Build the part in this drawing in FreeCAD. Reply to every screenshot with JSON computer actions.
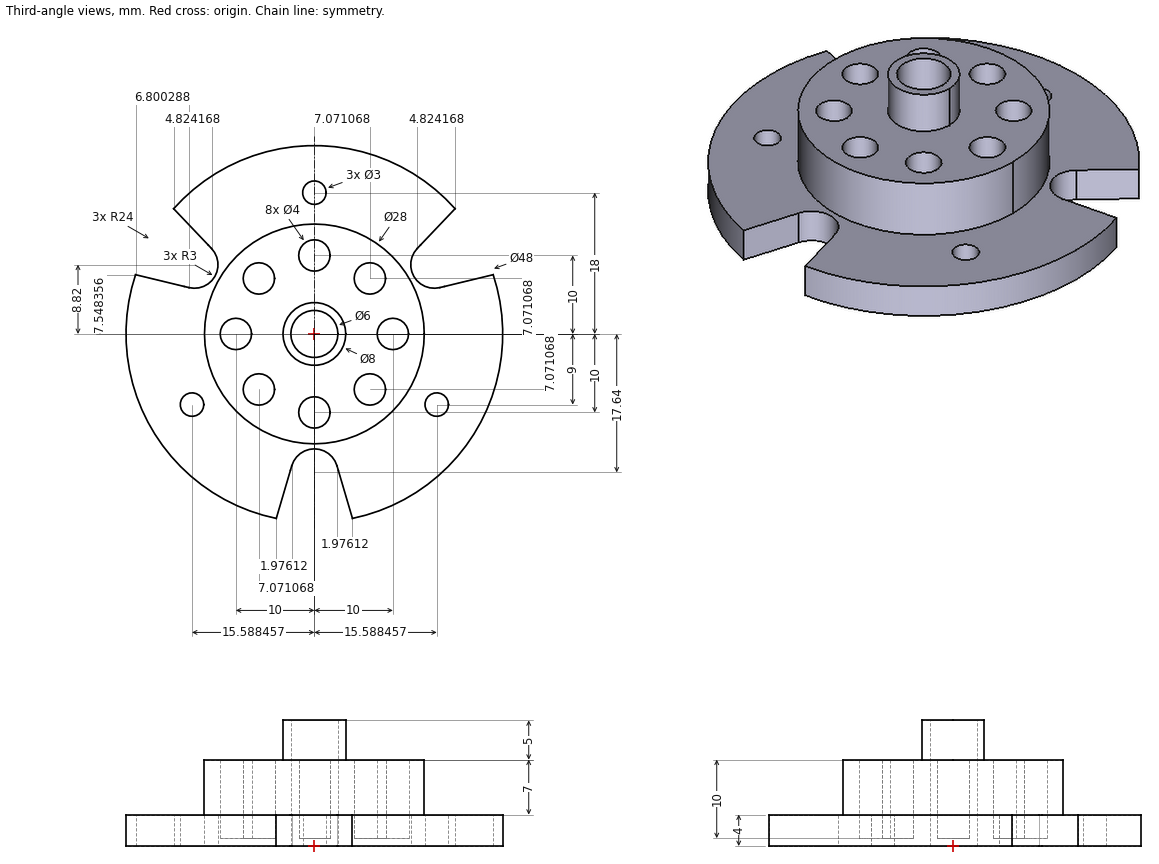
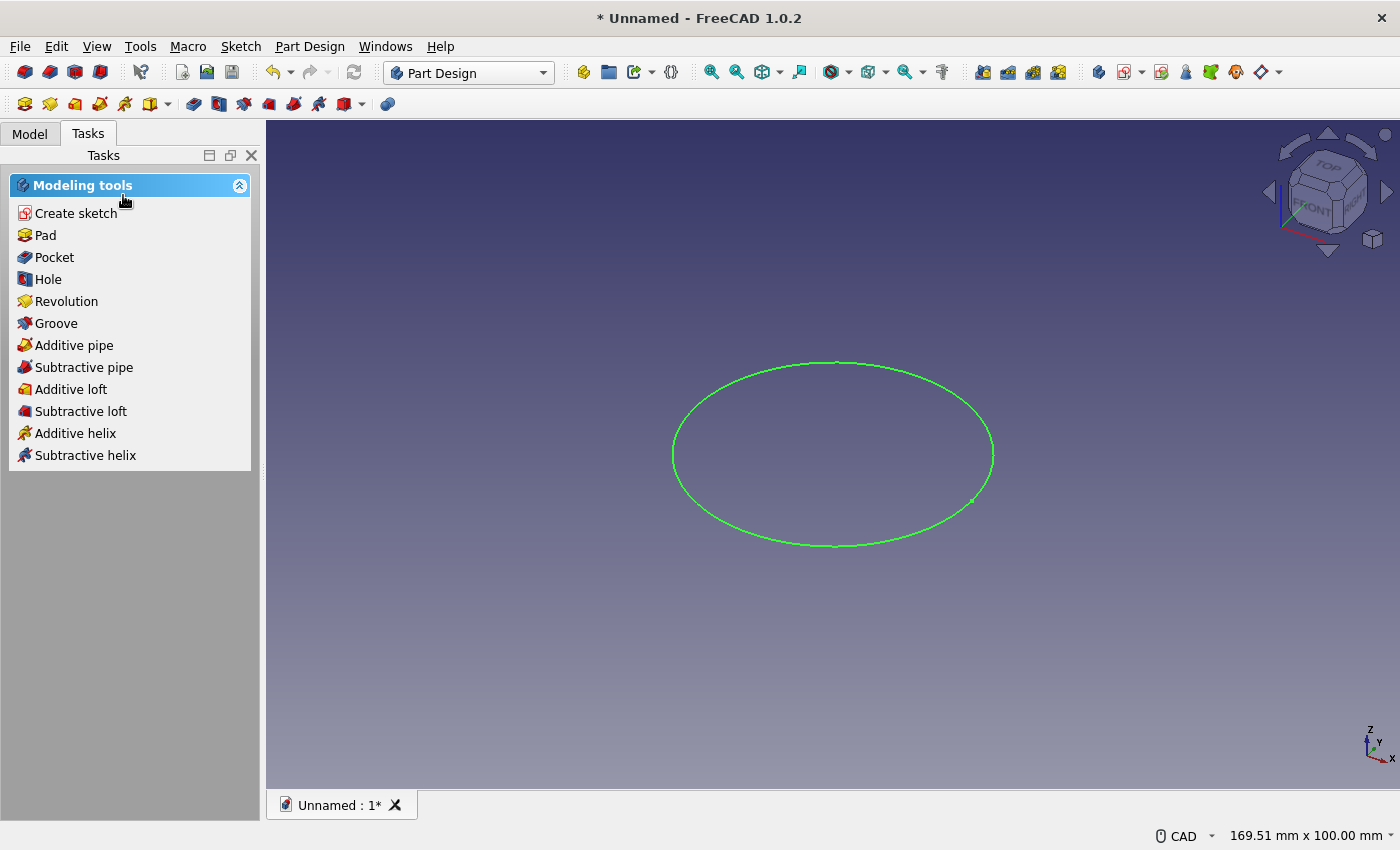
{"action": "left_click", "coordinate": [25, 104]}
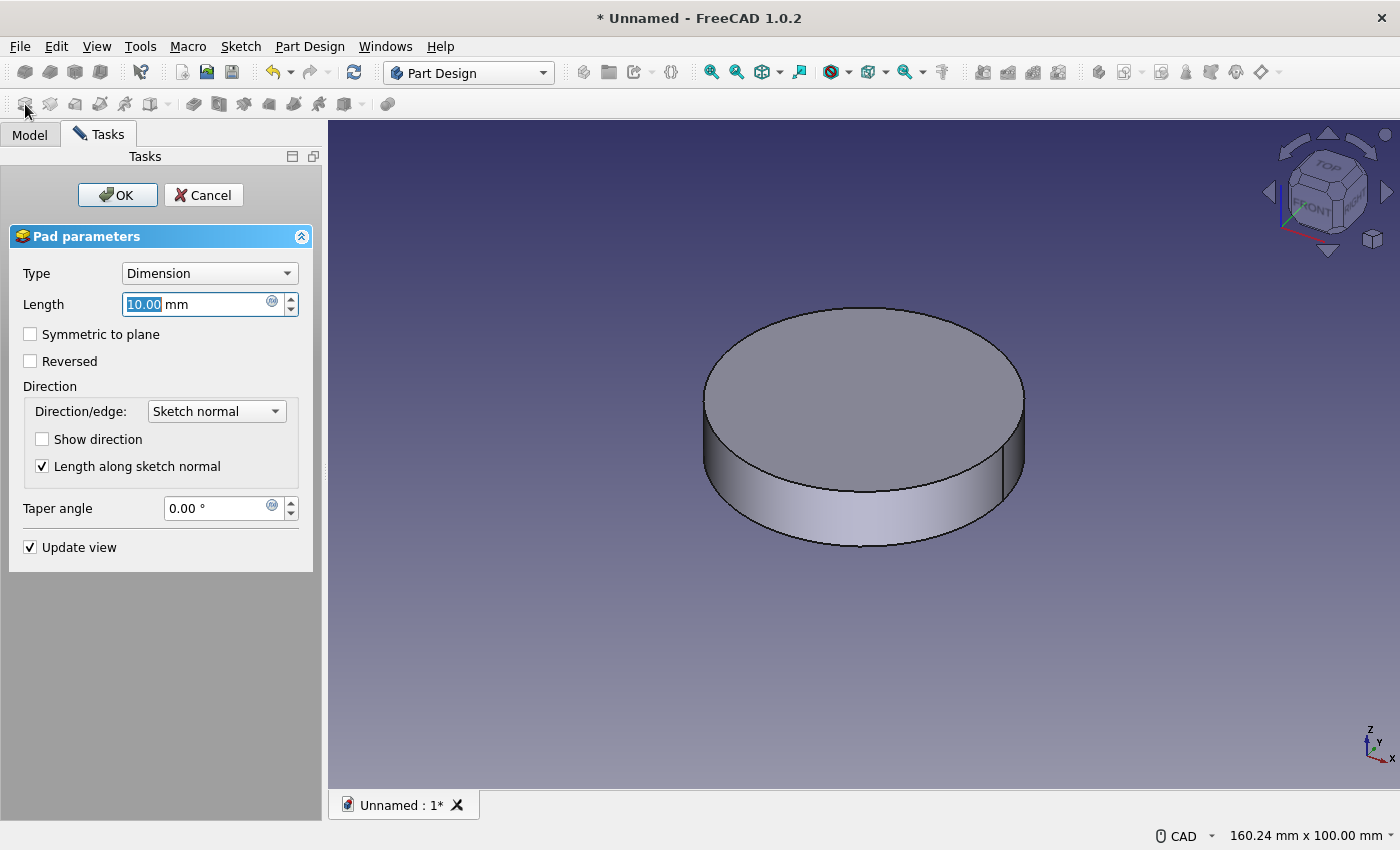
{"action": "type", "text": "4"}
{"action": "key", "text": "Tab"}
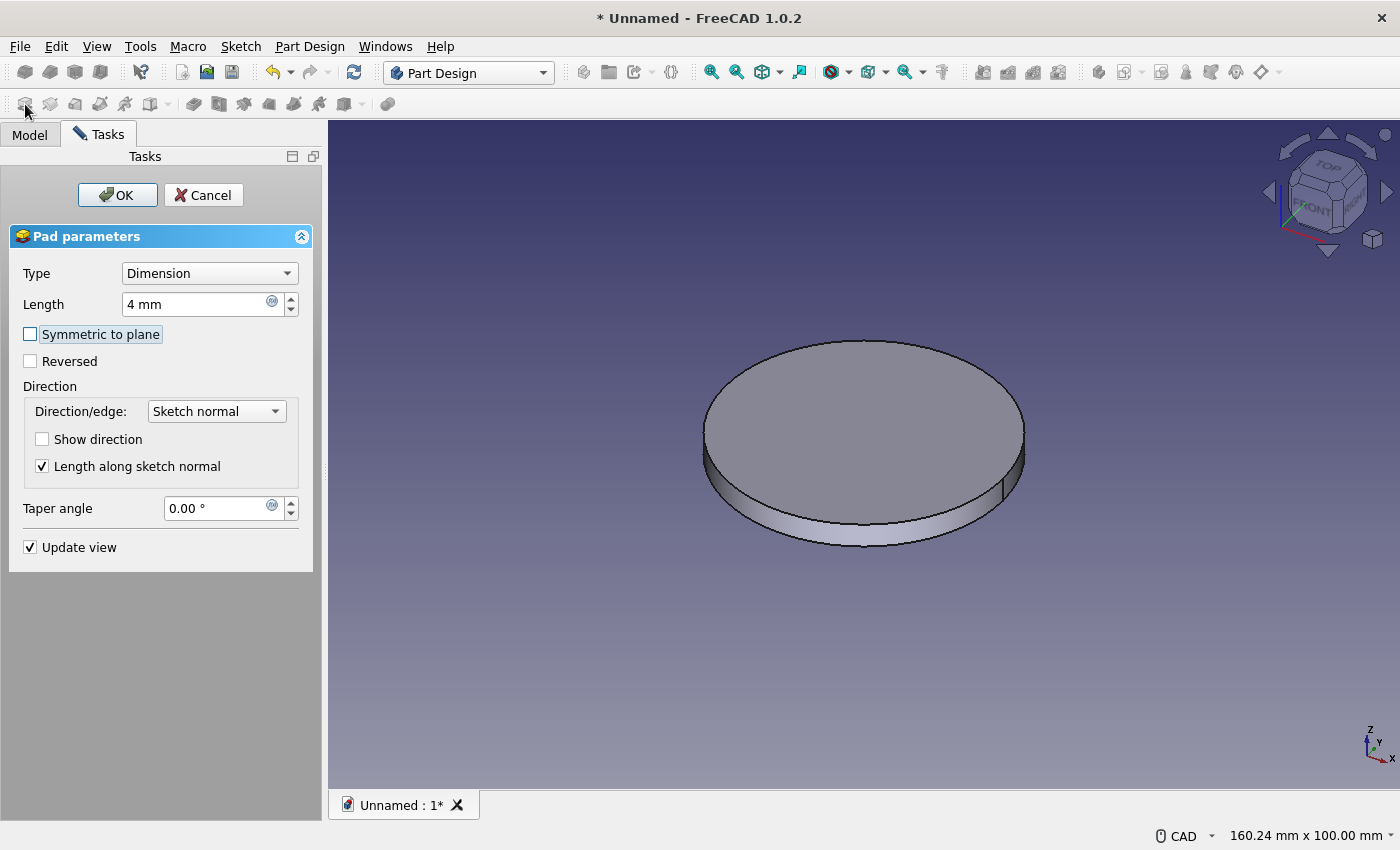
{"action": "left_click", "coordinate": [118, 195]}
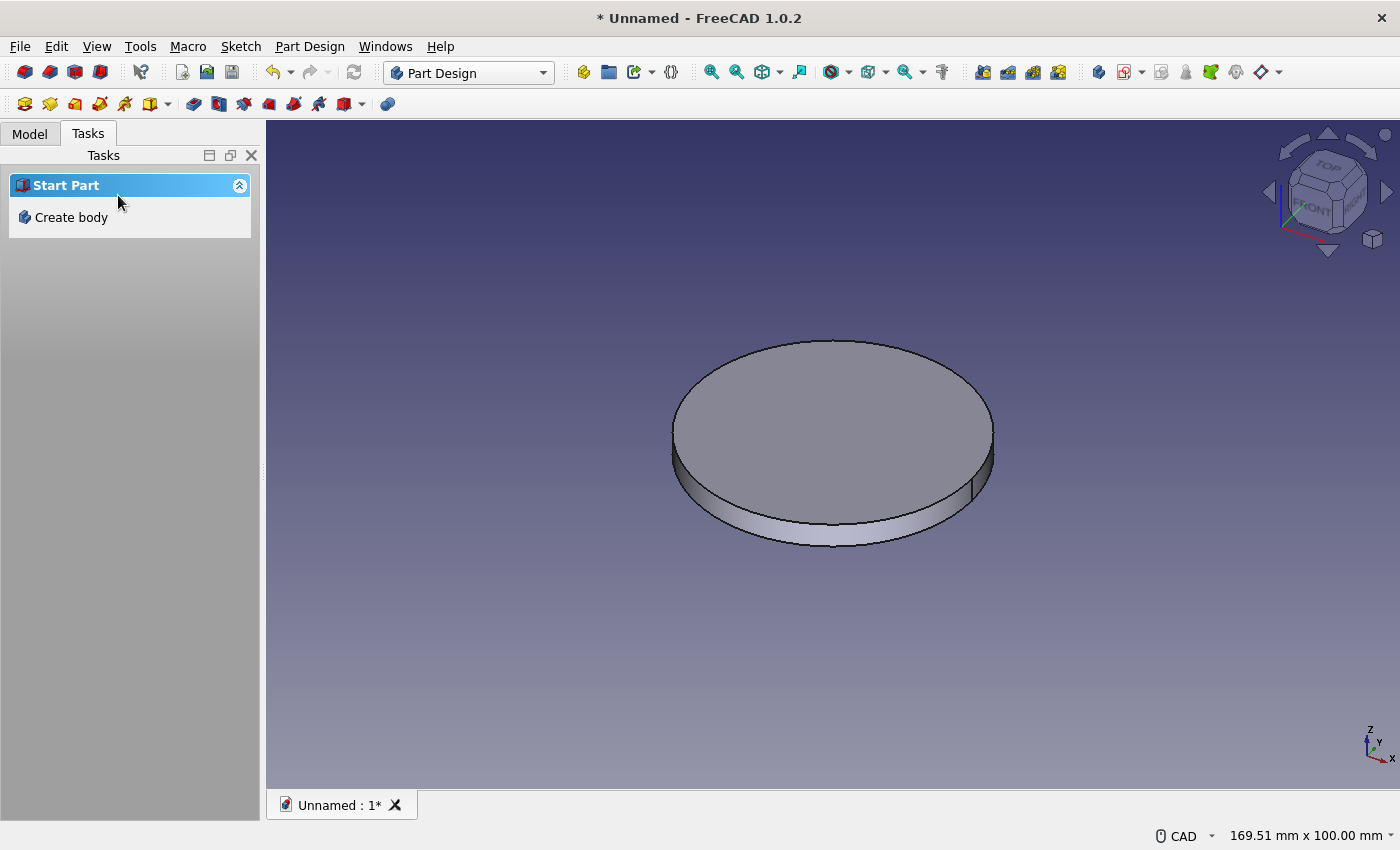
{"action": "key", "text": "v f"}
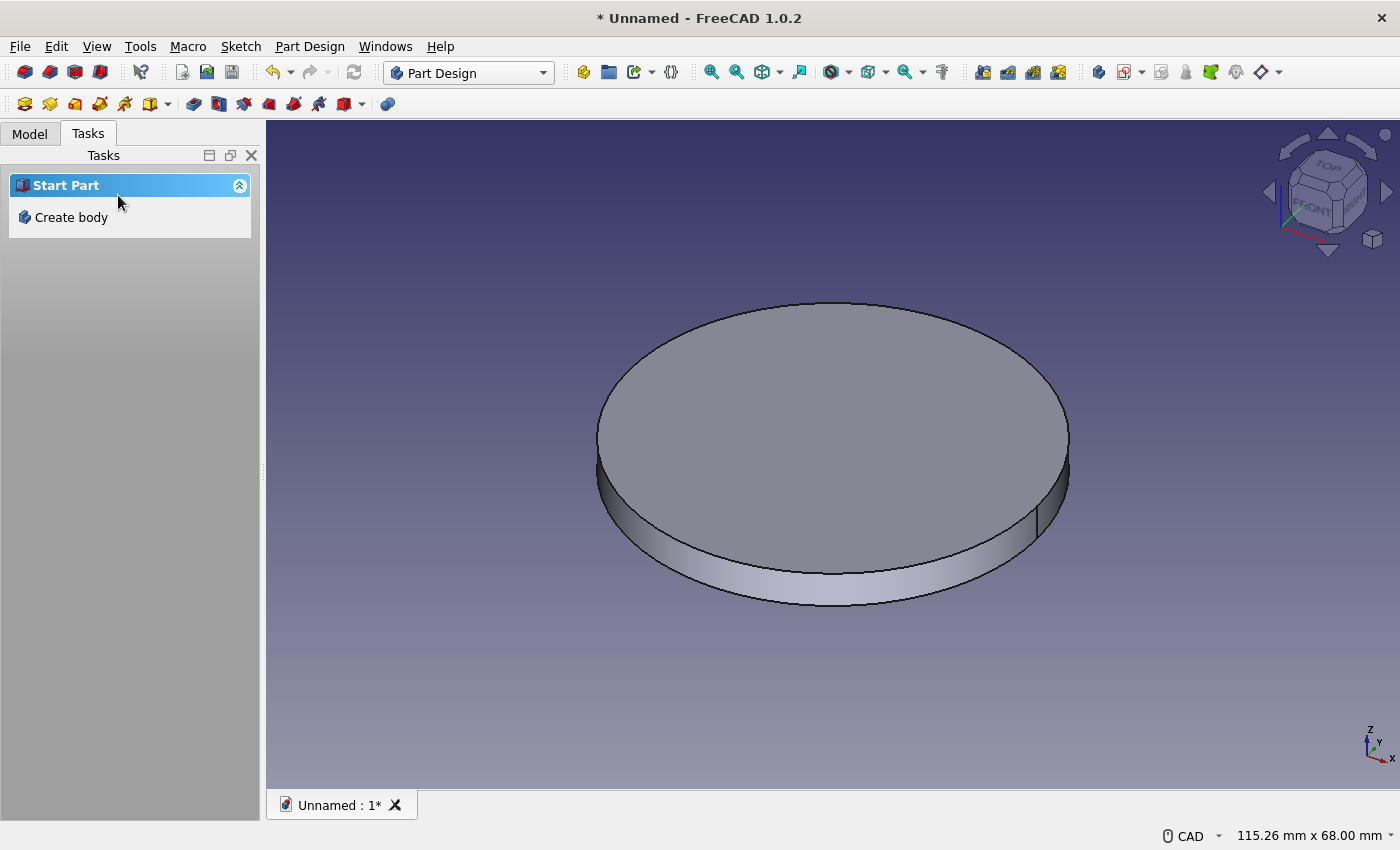
{"action": "left_click", "coordinate": [833, 437]}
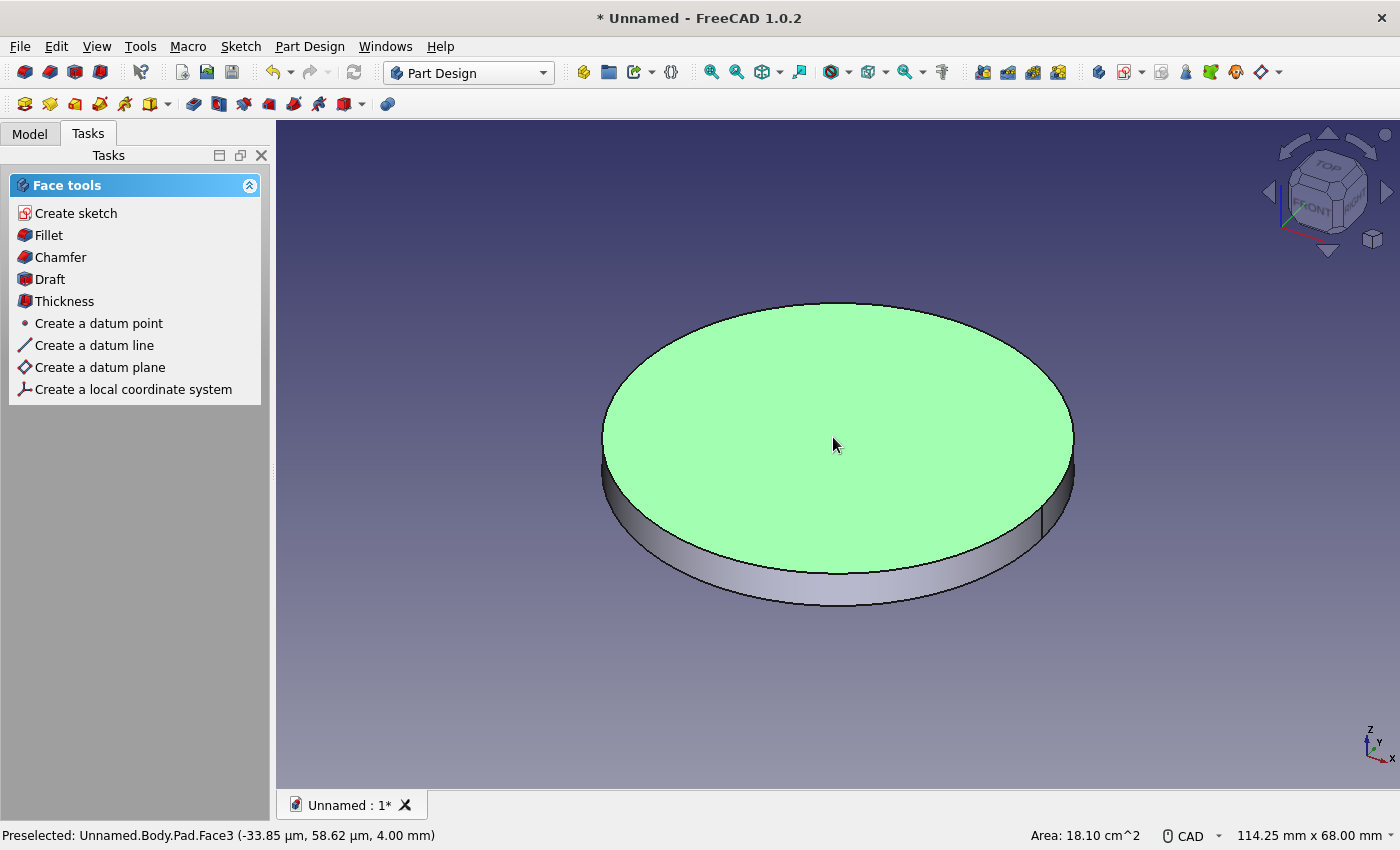
{"action": "left_click", "coordinate": [1124, 72]}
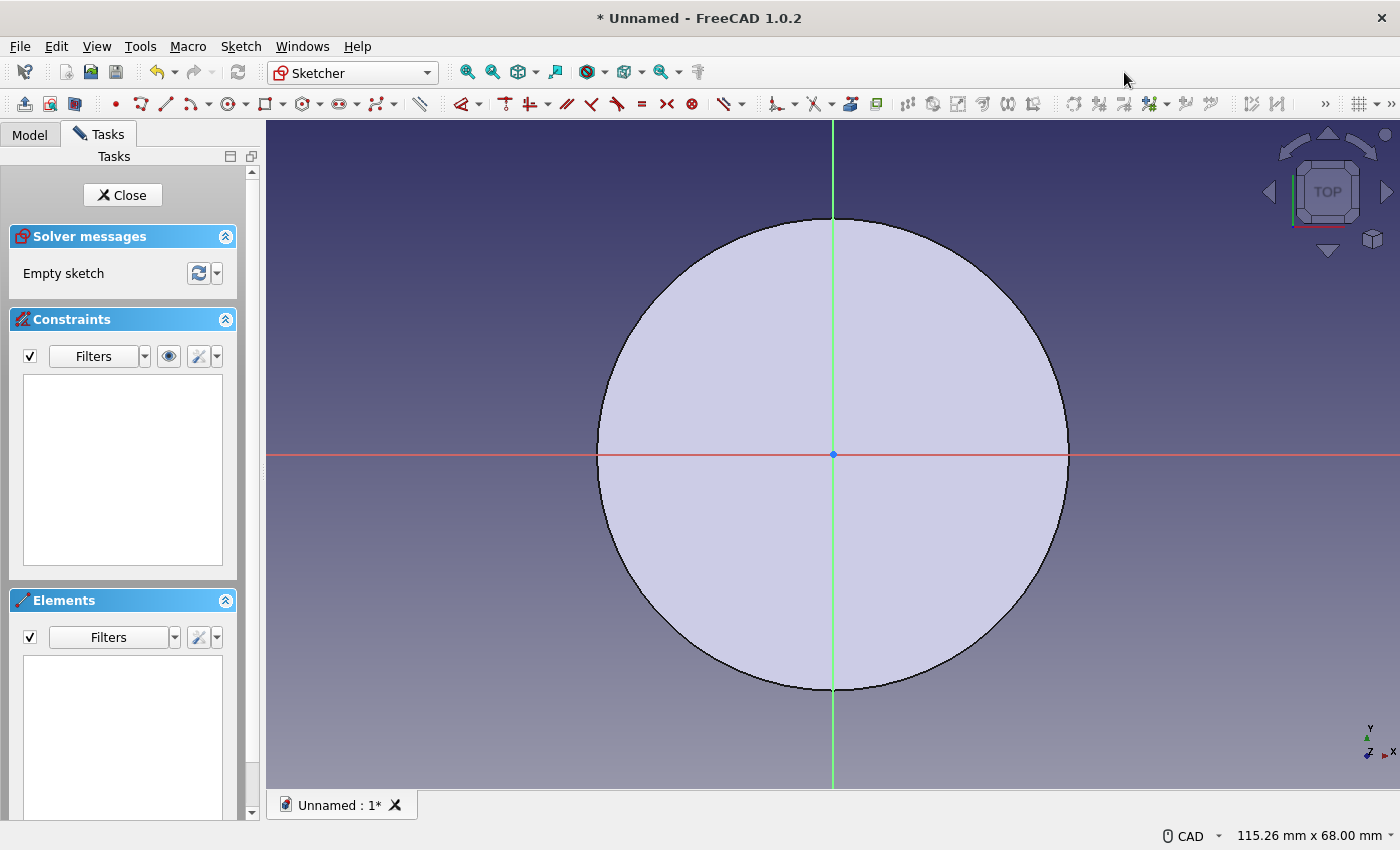
{"action": "scroll", "coordinate": [972, 455], "scroll_direction": "up", "scroll_amount": 2}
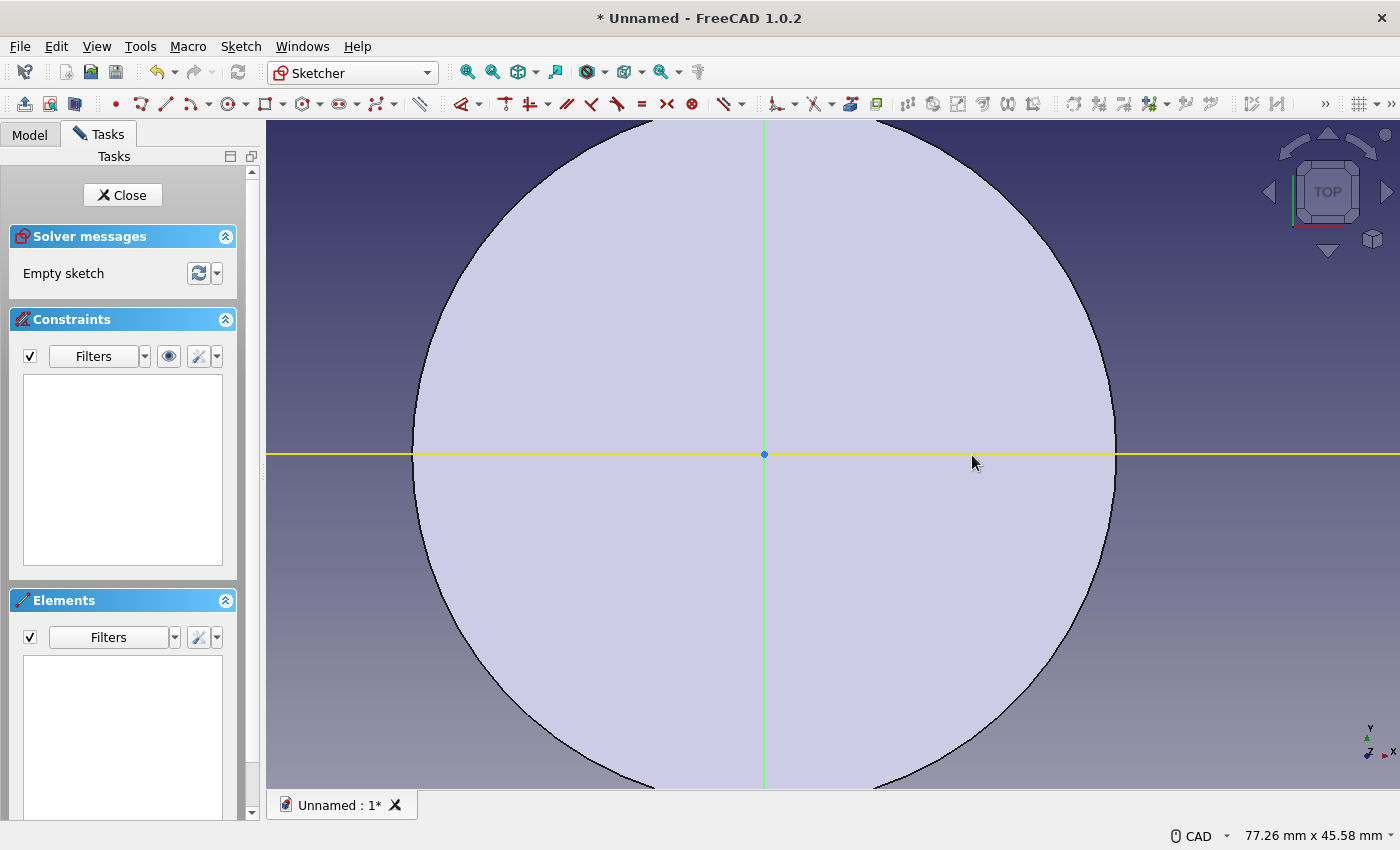
{"action": "key", "text": "g c"}